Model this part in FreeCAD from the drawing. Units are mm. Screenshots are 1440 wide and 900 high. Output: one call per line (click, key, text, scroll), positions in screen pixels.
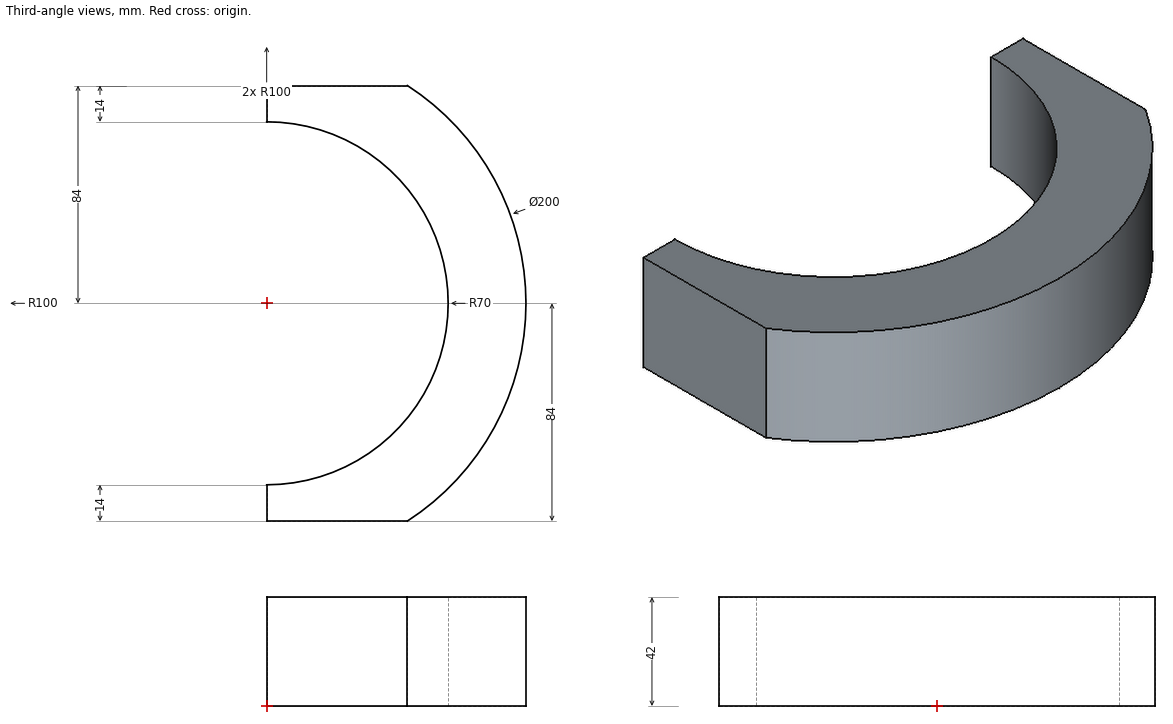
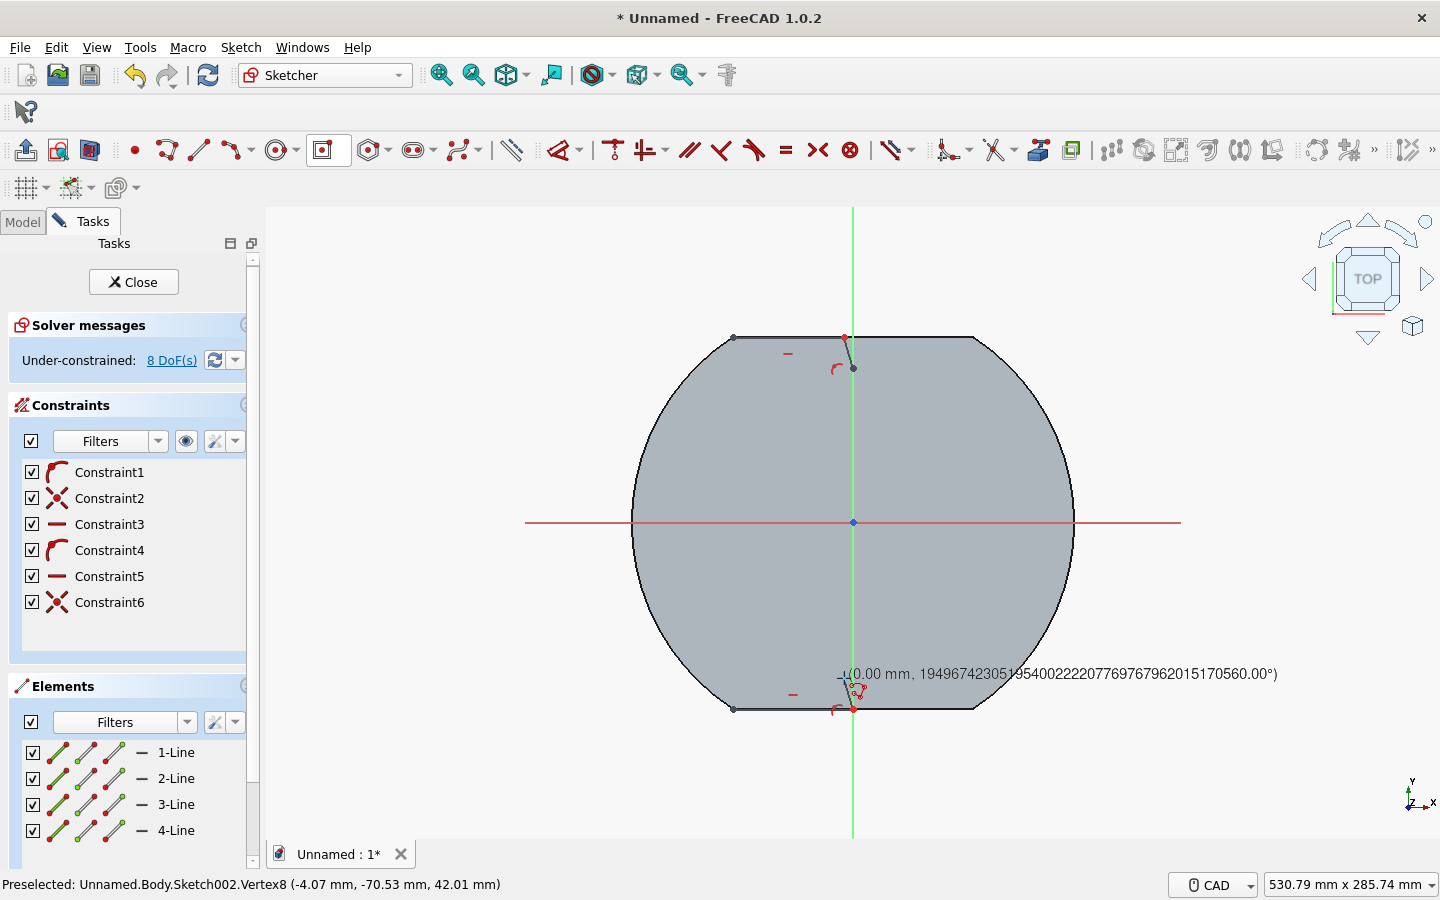
click(232, 150)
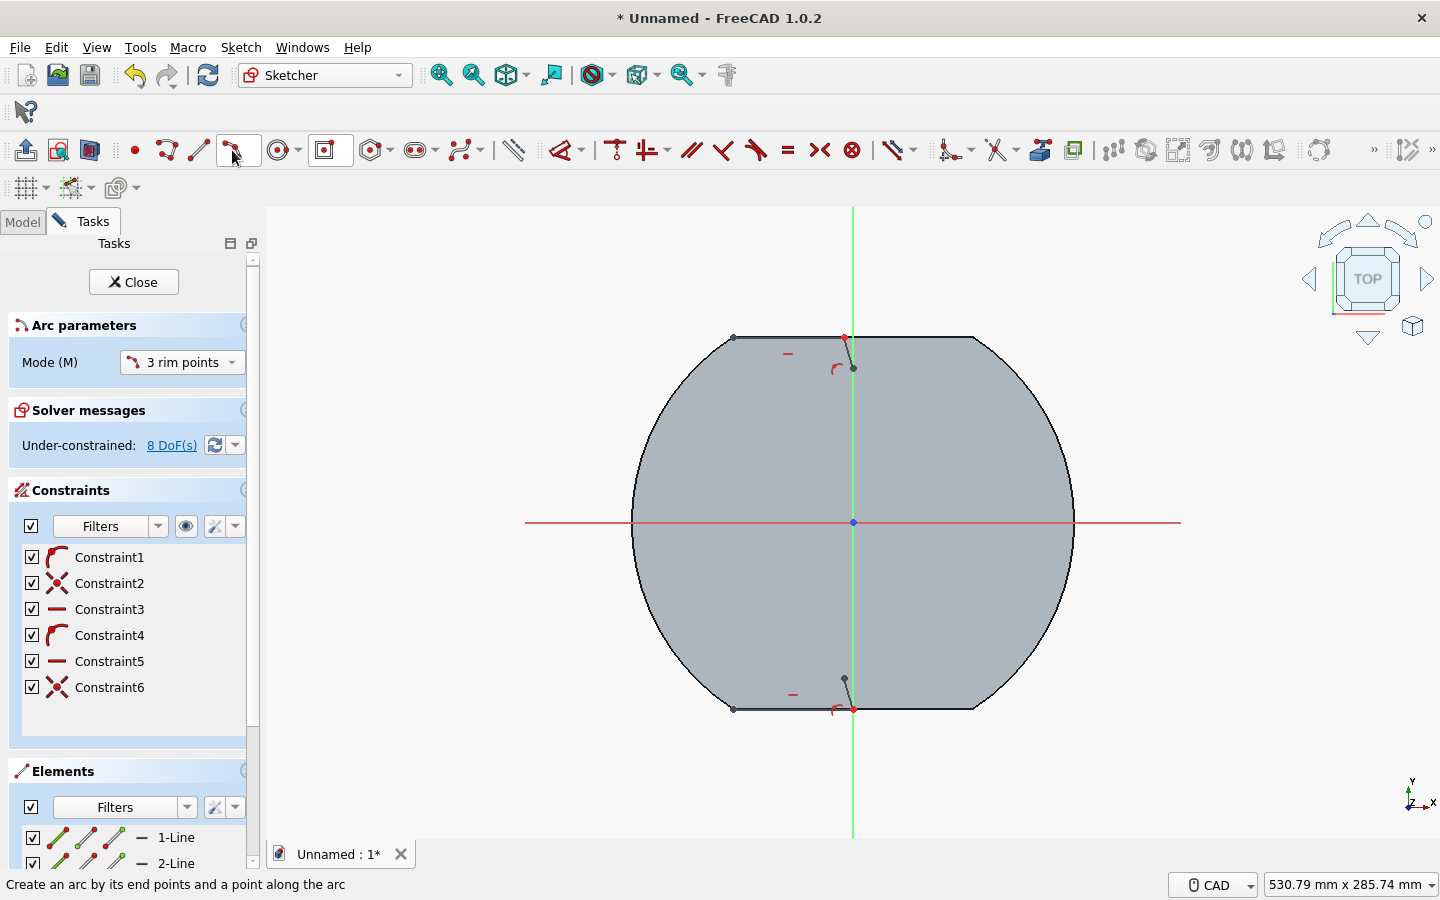
click(733, 338)
click(733, 710)
click(636, 479)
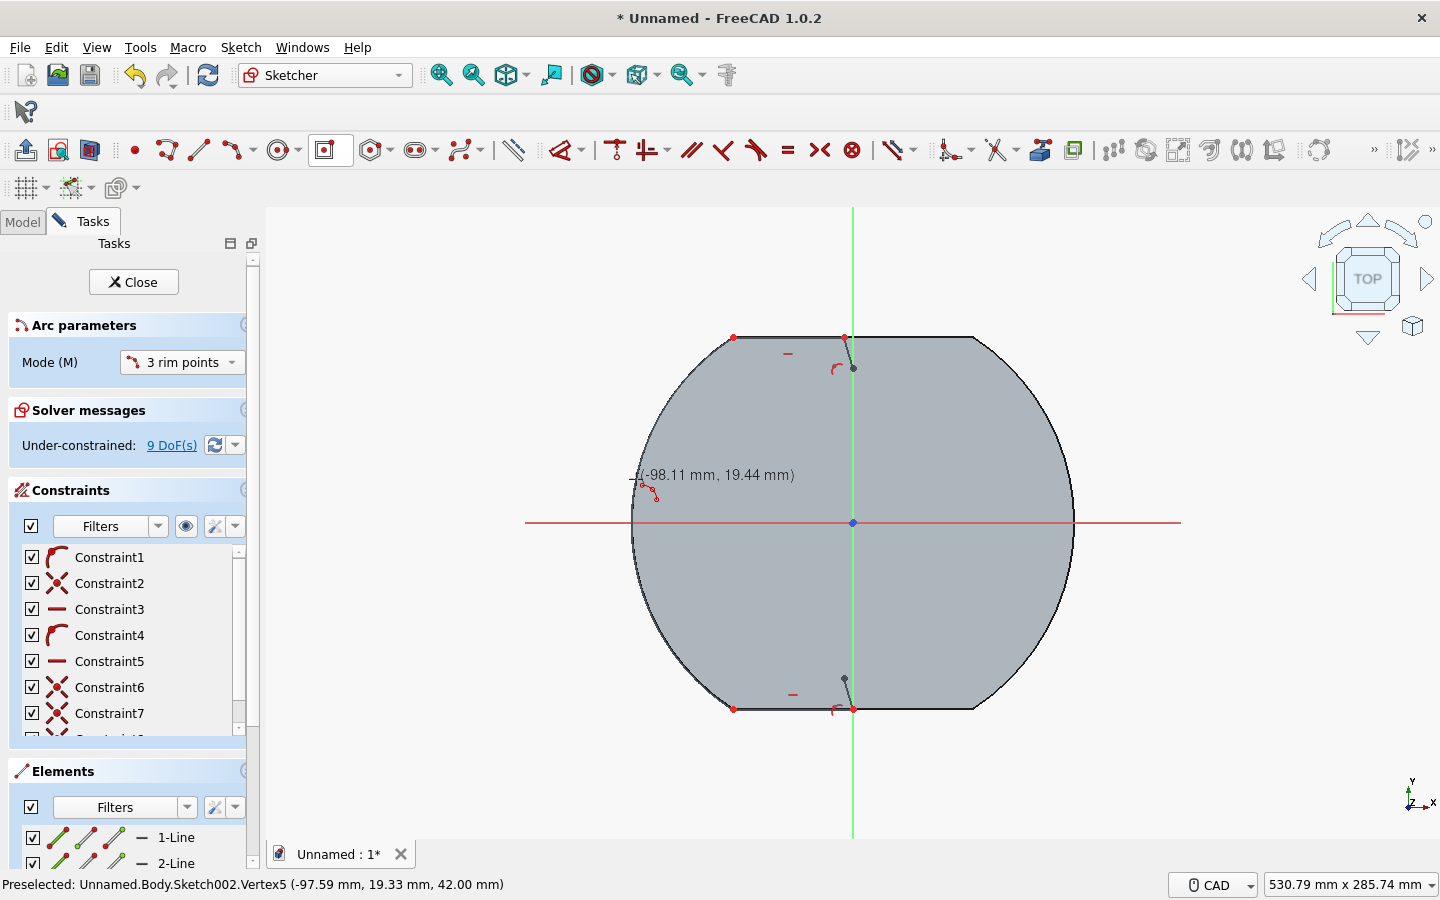
click(844, 679)
click(853, 369)
click(1000, 571)
key(Escape)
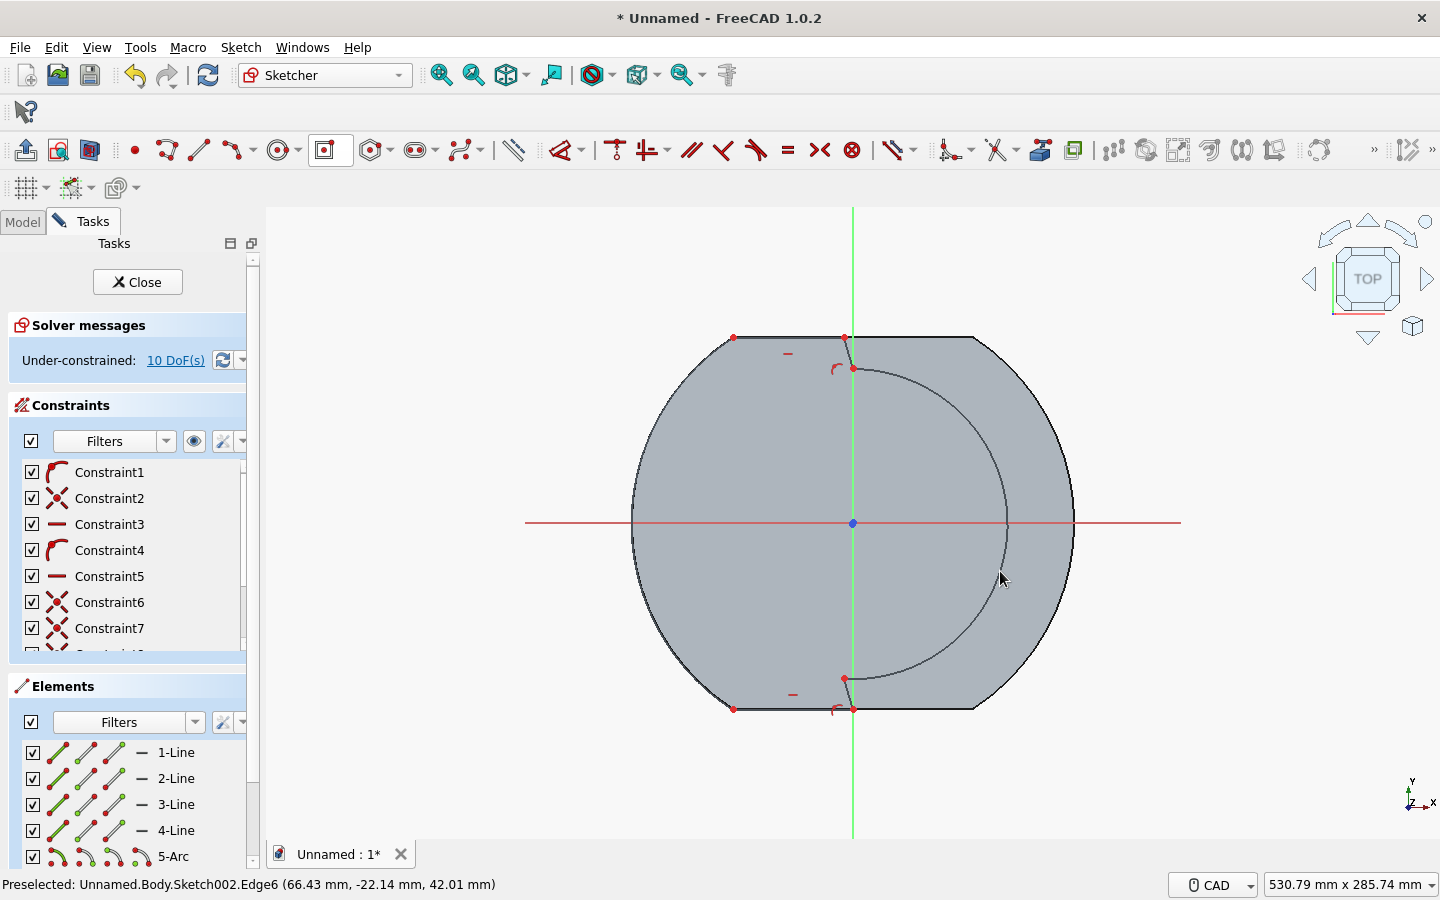
scroll(850, 360, up, 2)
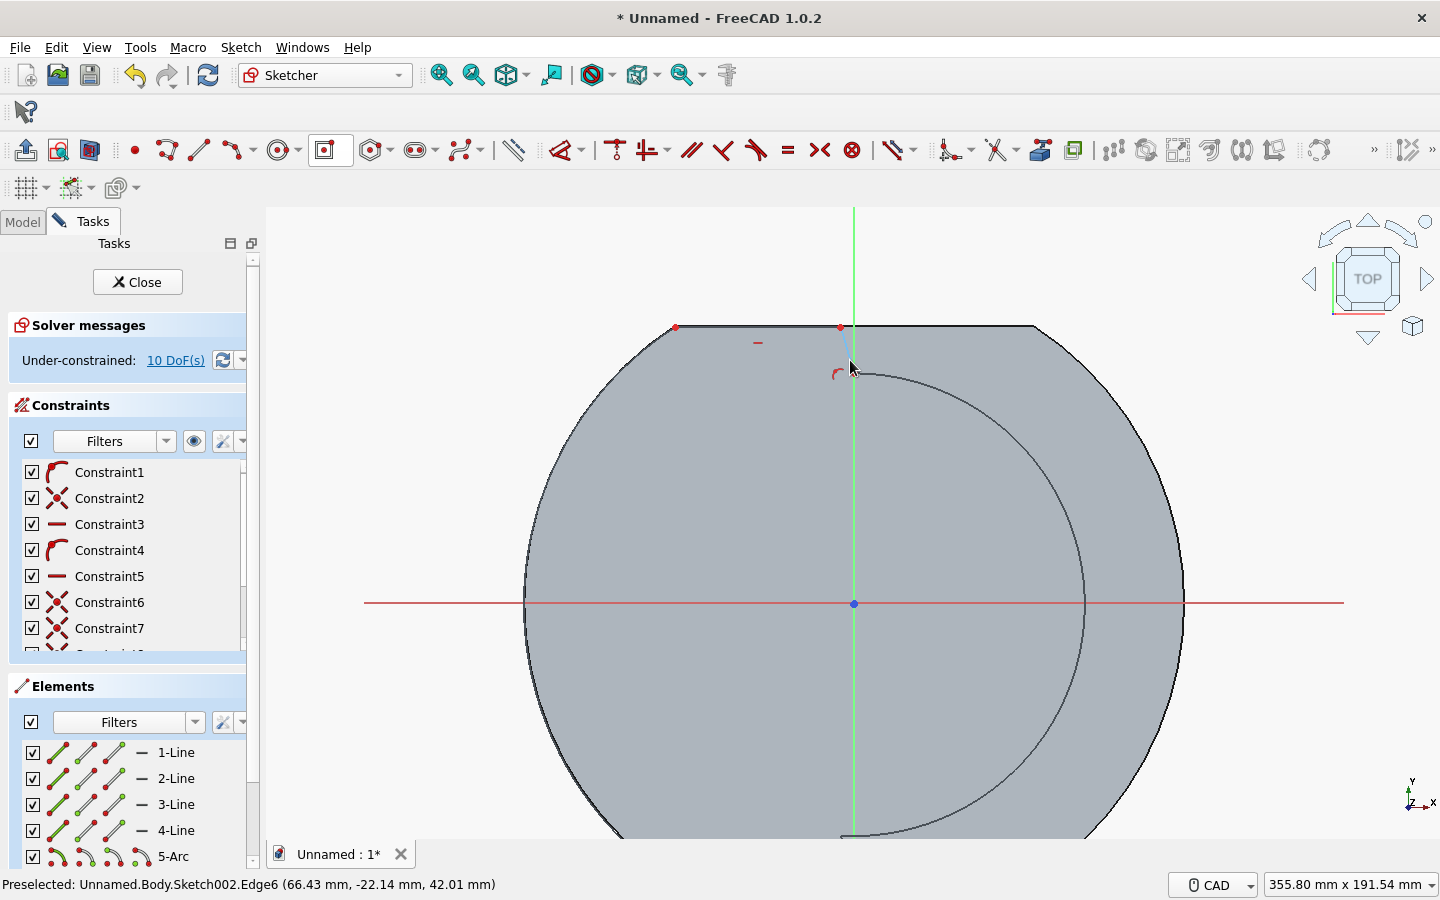
click(850, 359)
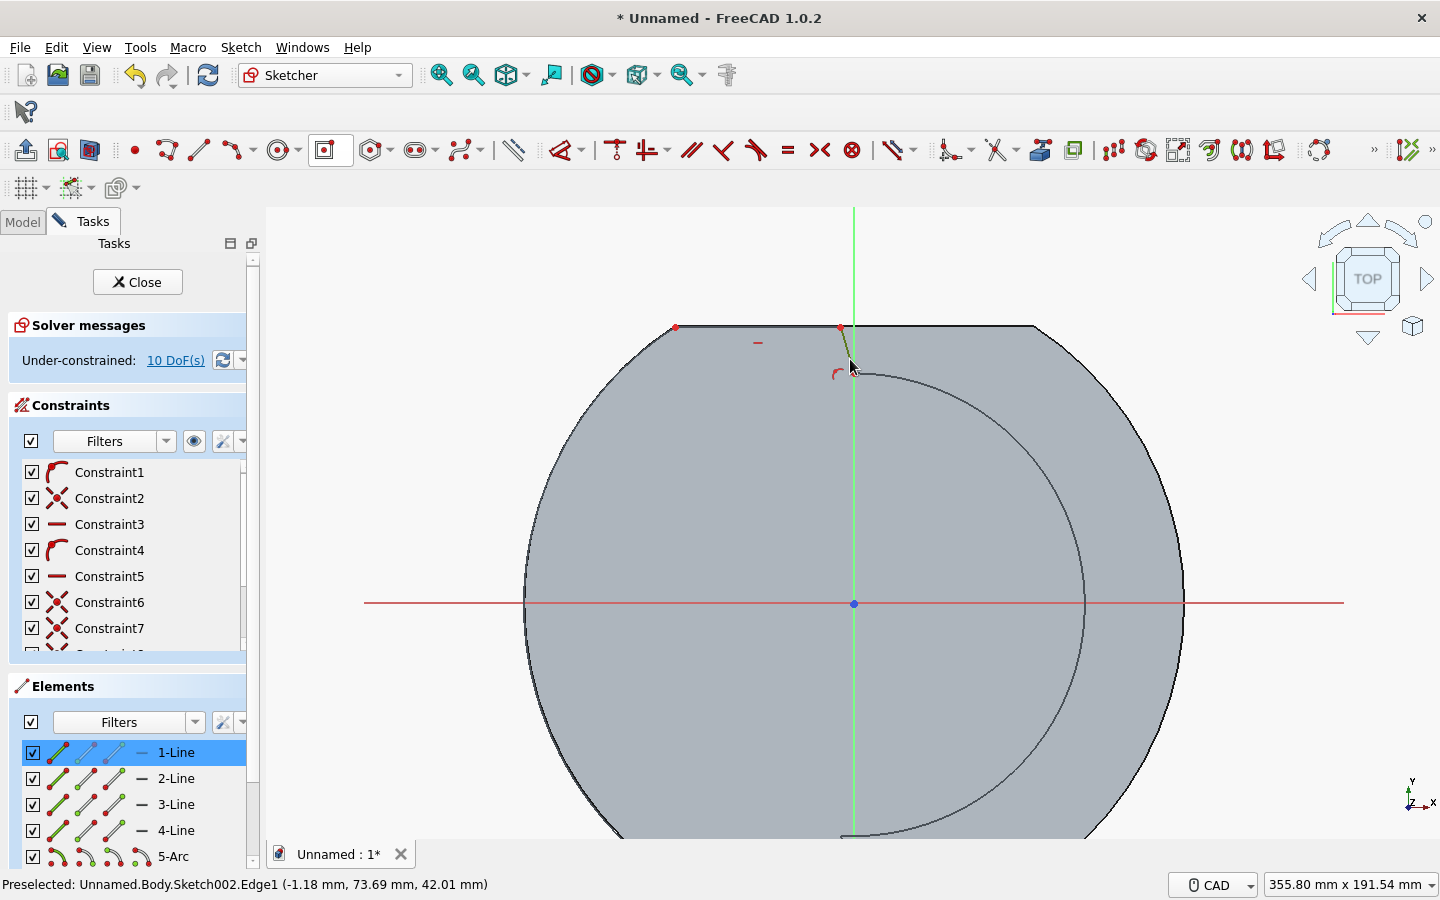
key(v)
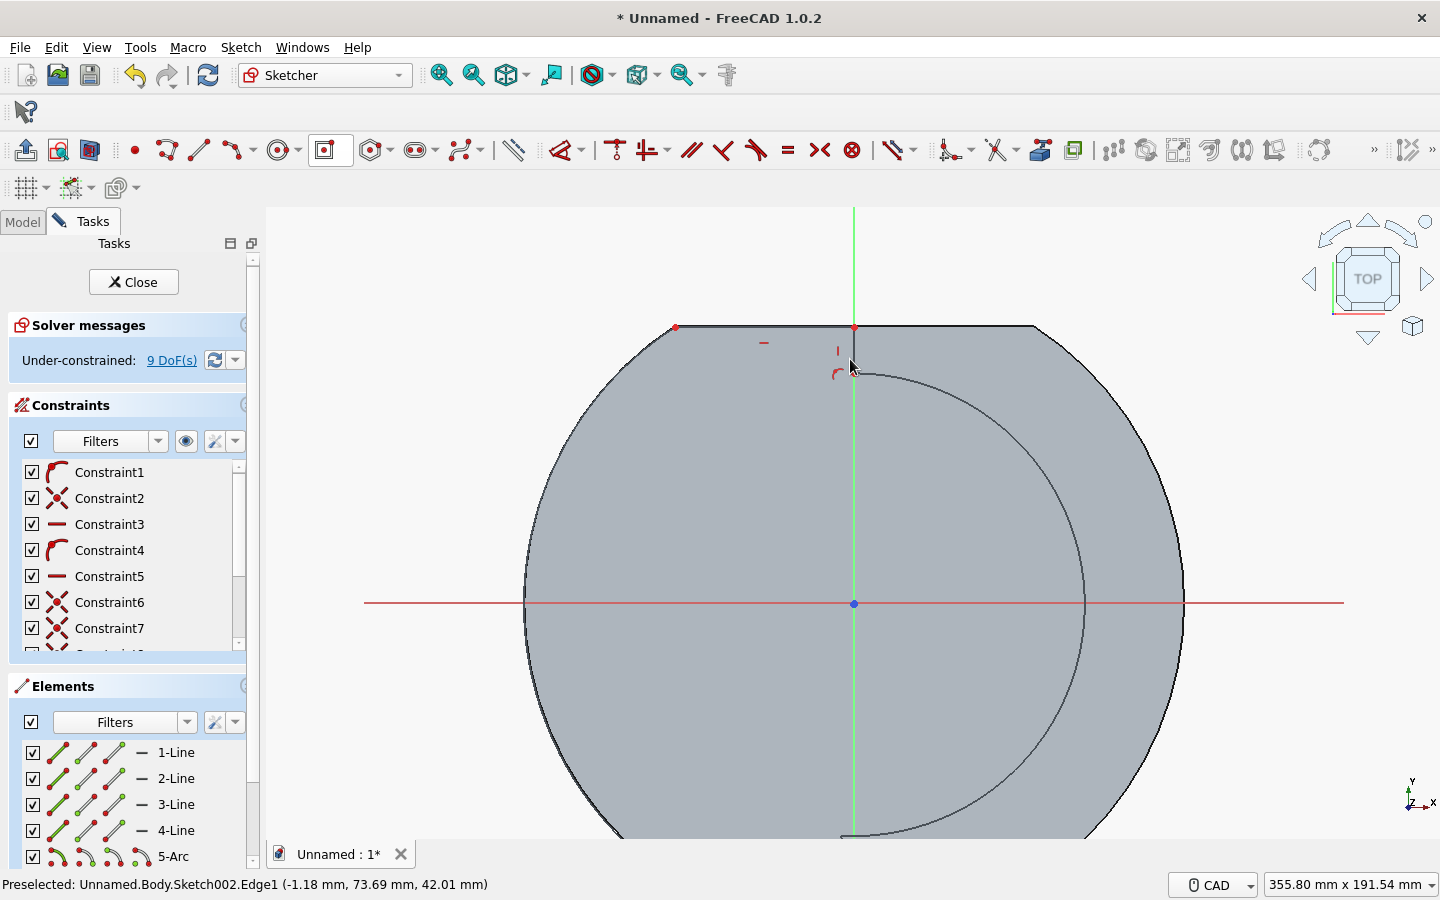
scroll(743, 360, down, 2)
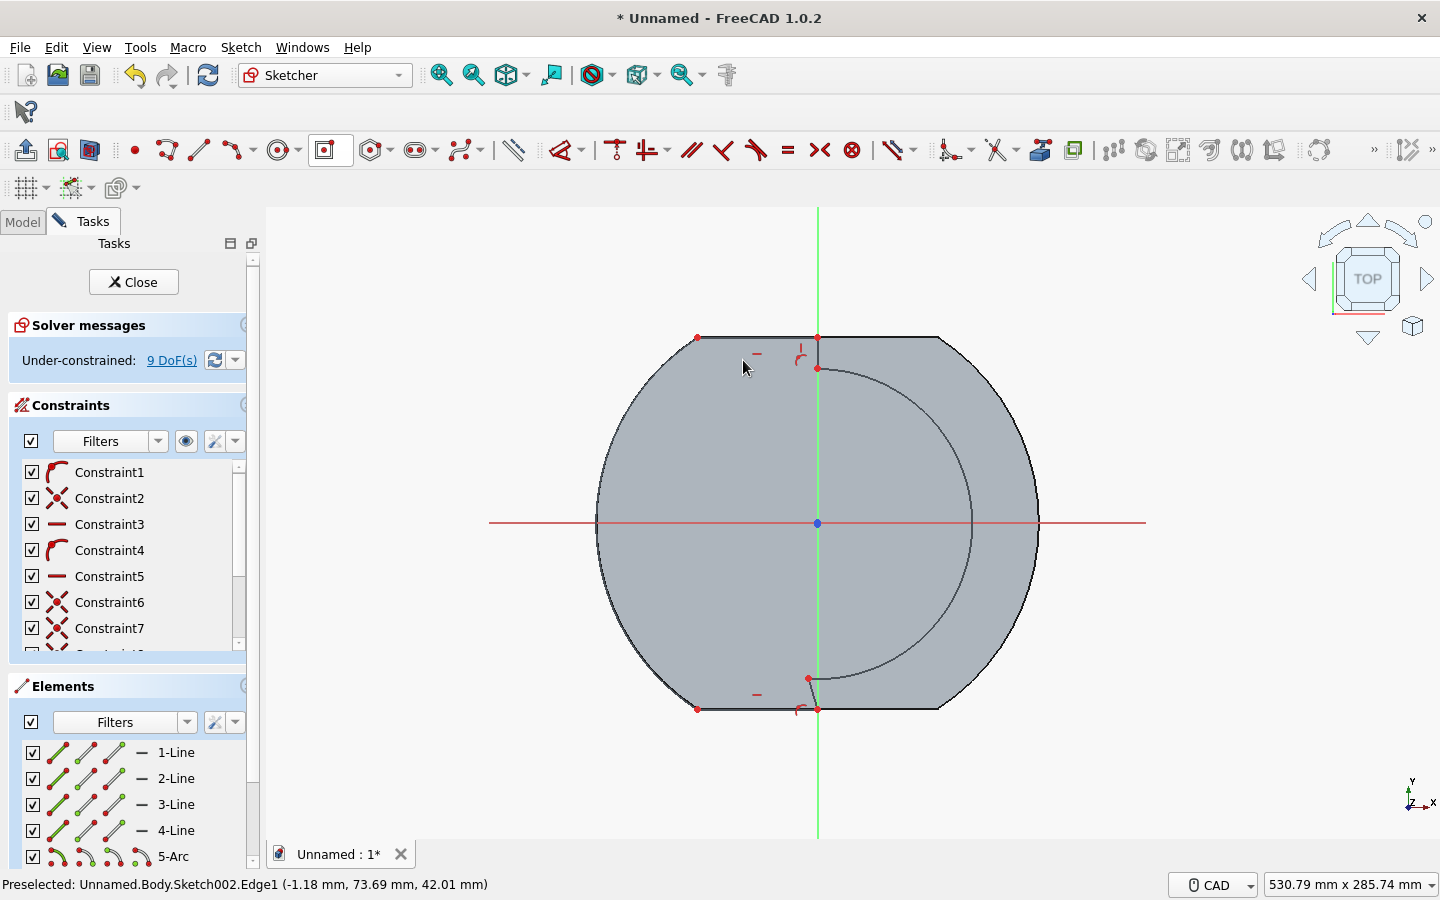
scroll(811, 688, up, 4)